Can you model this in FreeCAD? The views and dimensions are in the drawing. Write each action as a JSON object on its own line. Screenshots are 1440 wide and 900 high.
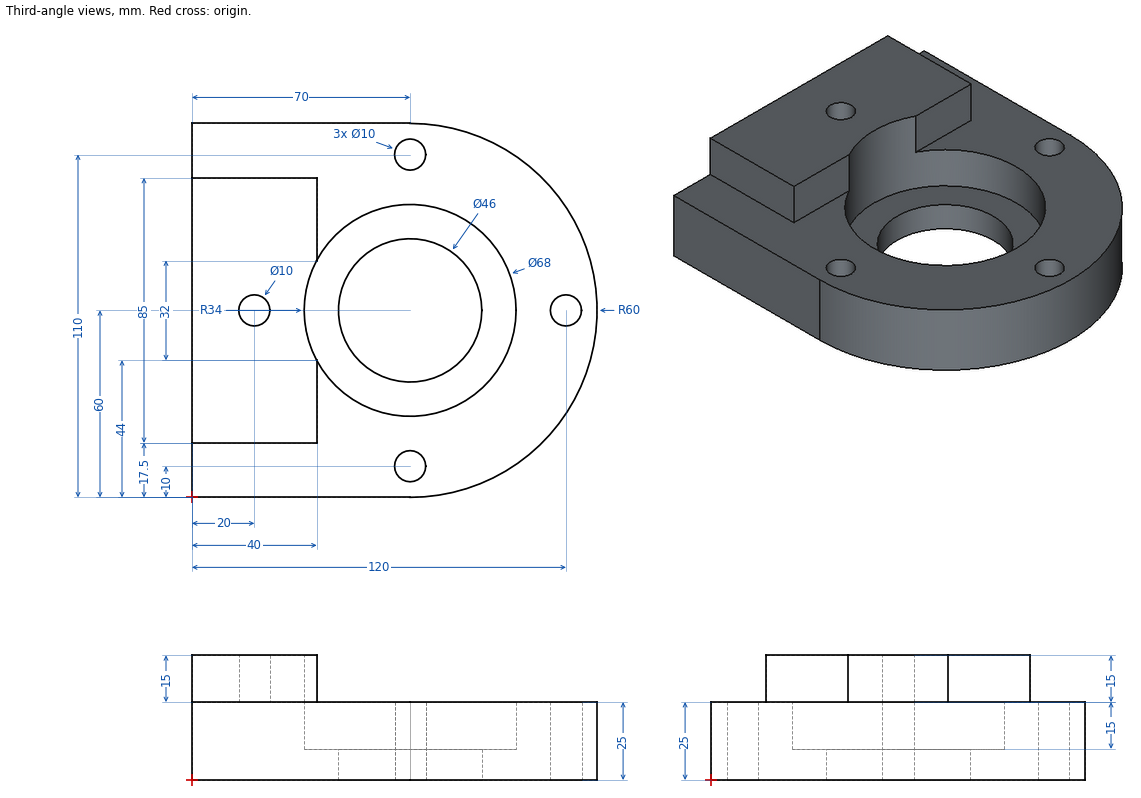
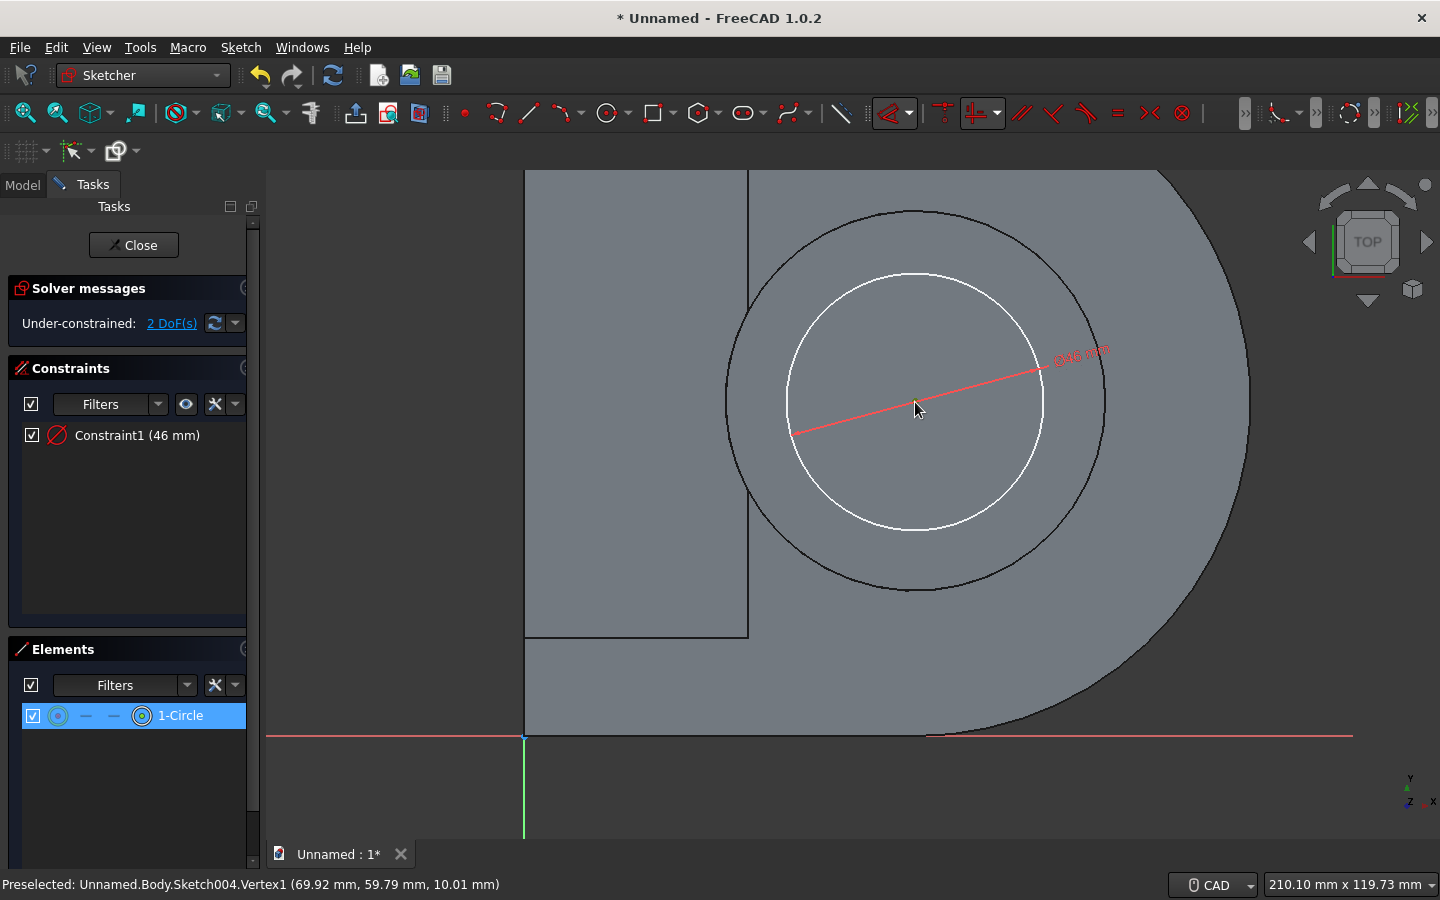
{"action": "key", "text": "l"}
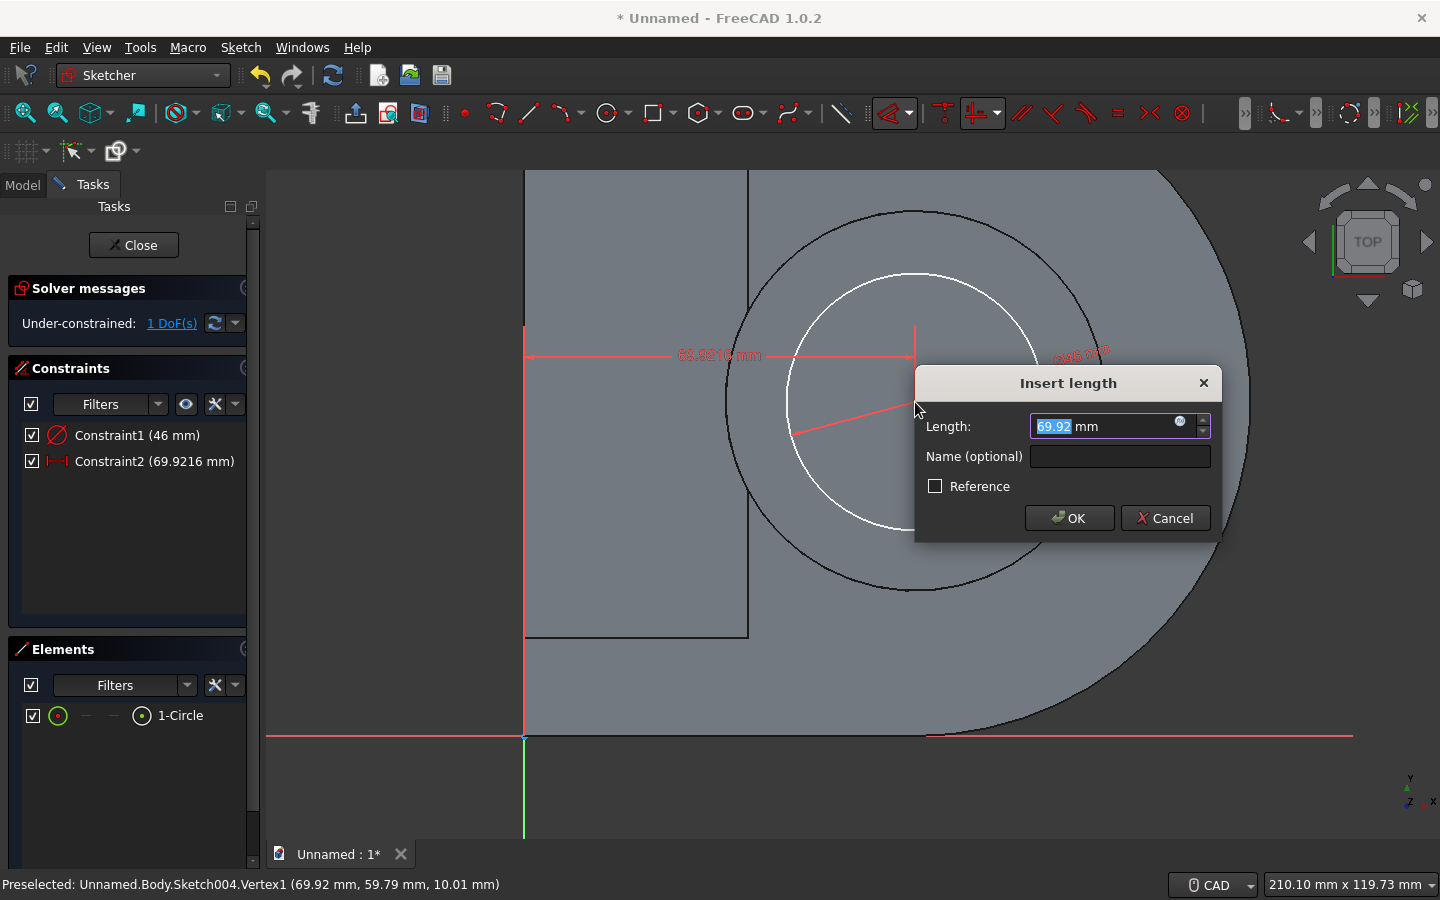
{"action": "type", "text": "70"}
{"action": "key", "text": "Return"}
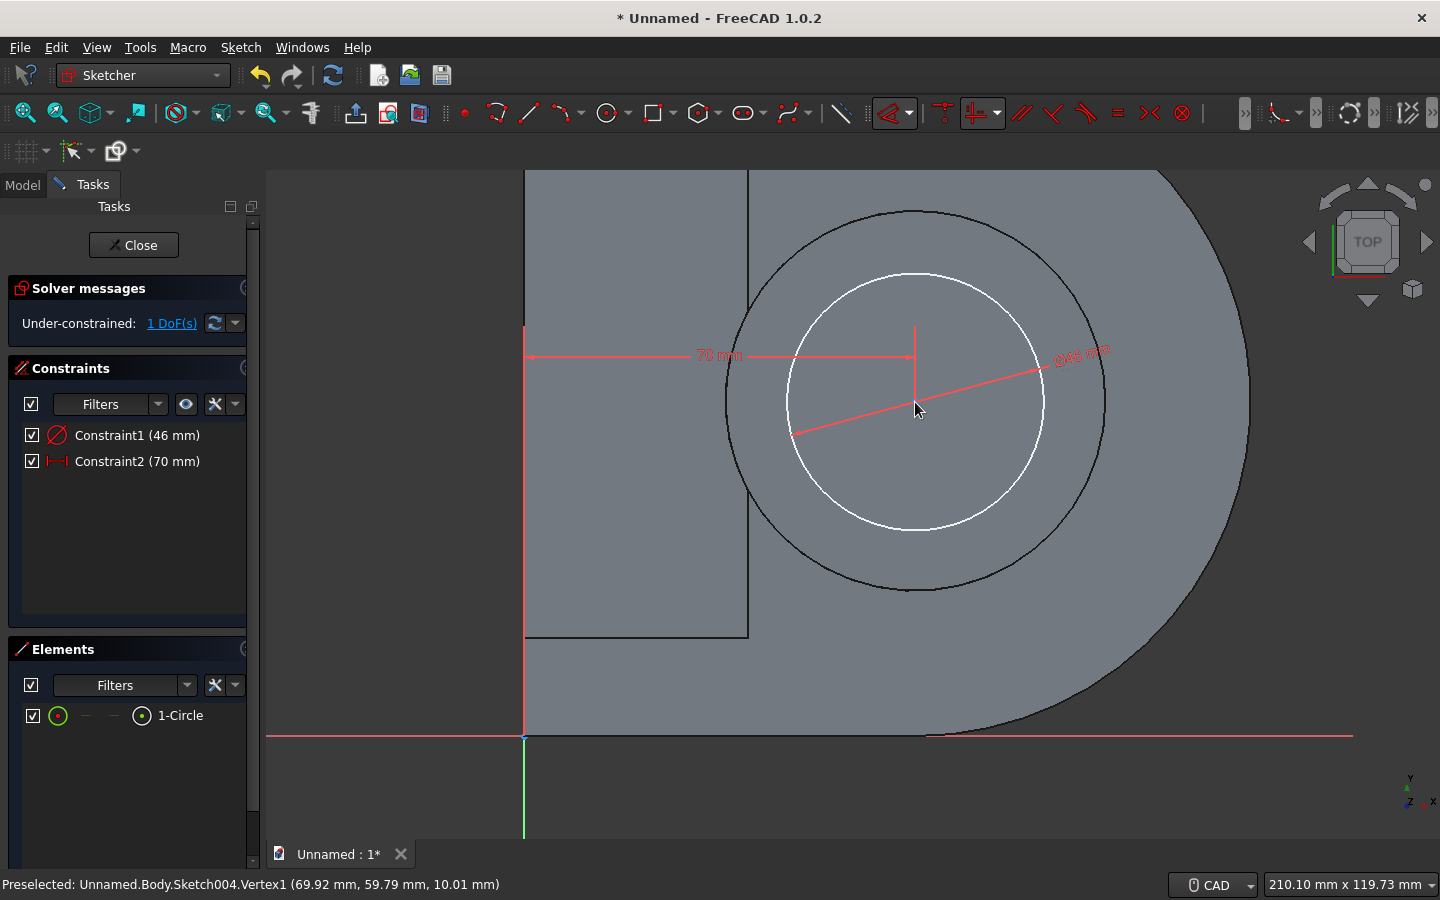
{"action": "left_click", "coordinate": [915, 402]}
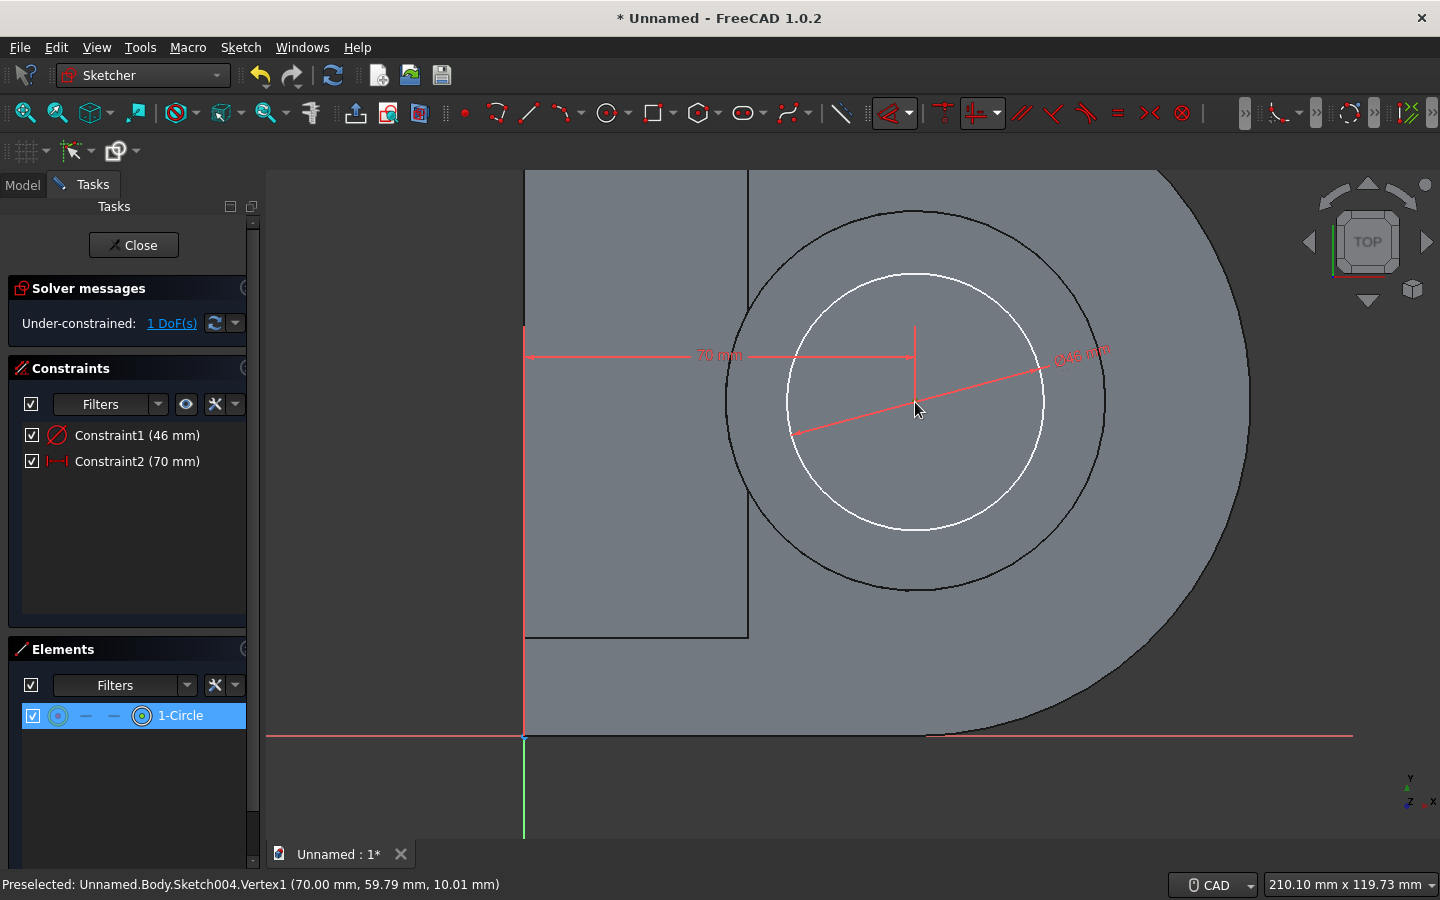
{"action": "left_click", "coordinate": [912, 114]}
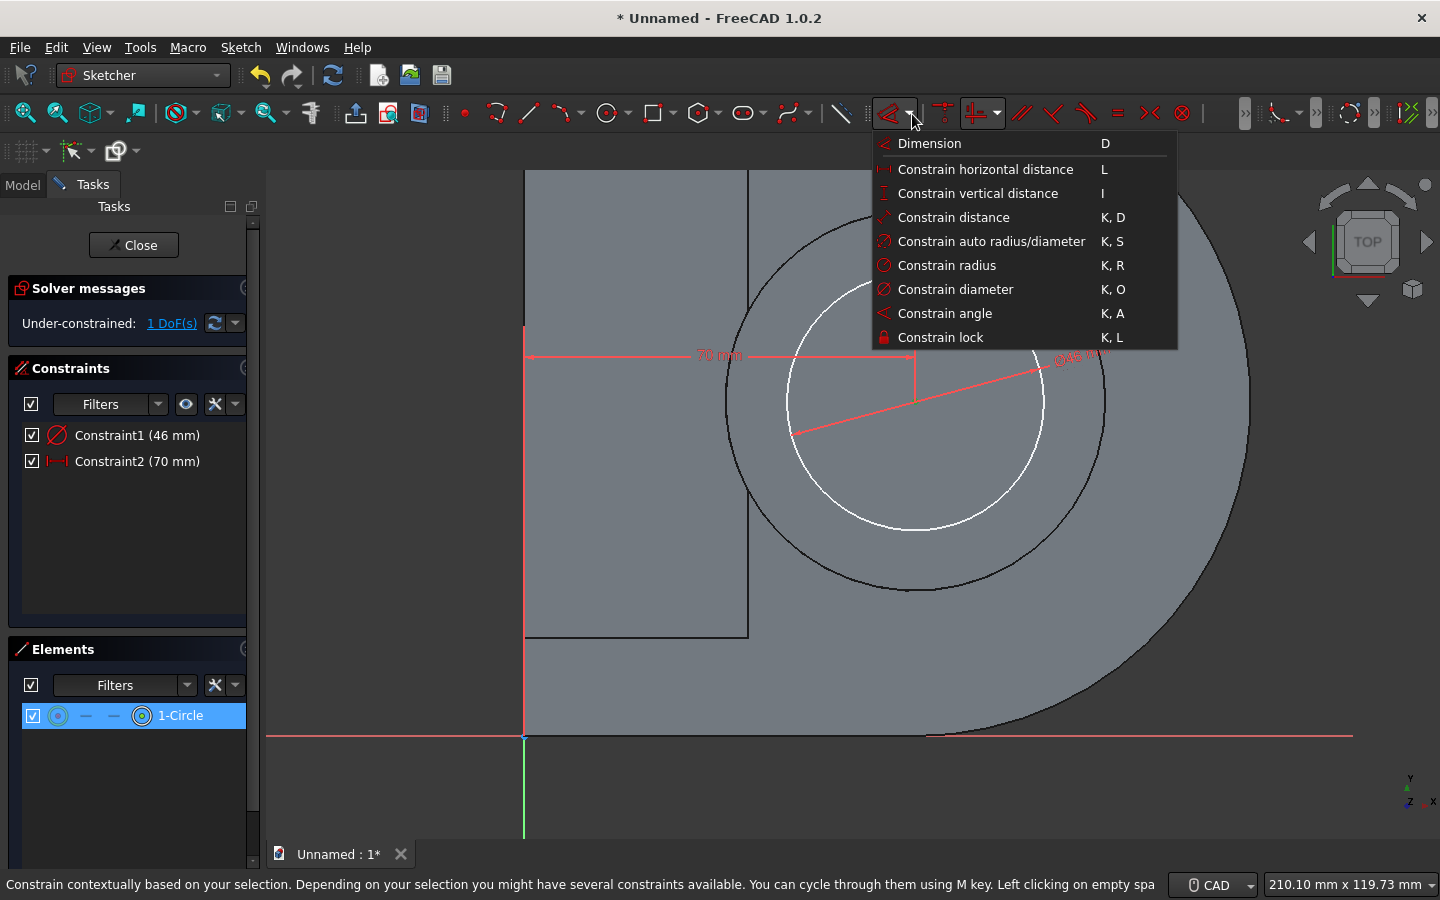
{"action": "left_click", "coordinate": [1025, 193]}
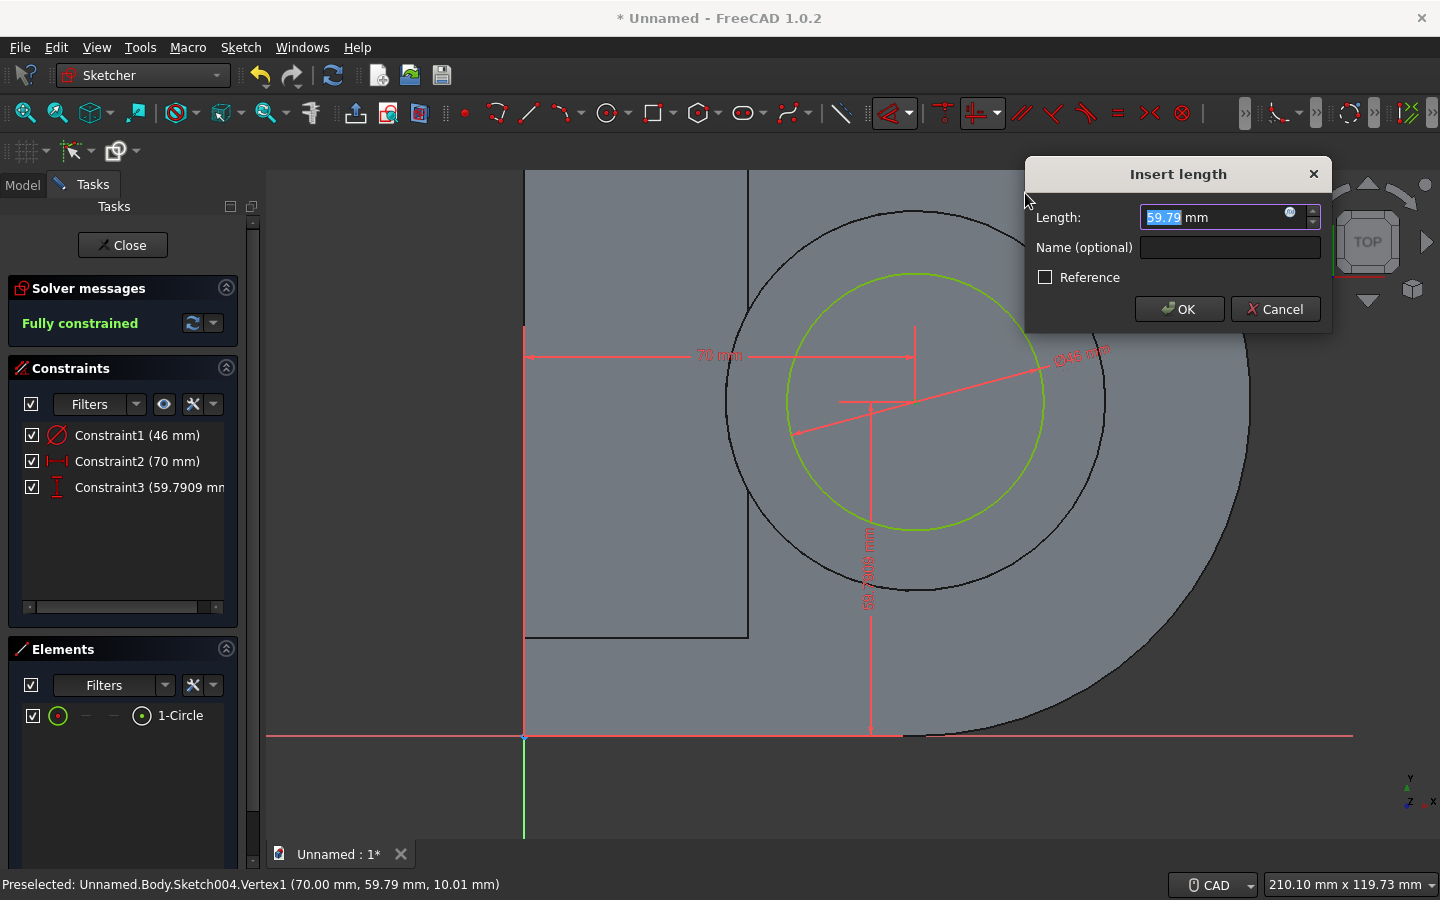
{"action": "type", "text": "60"}
{"action": "key", "text": "Return"}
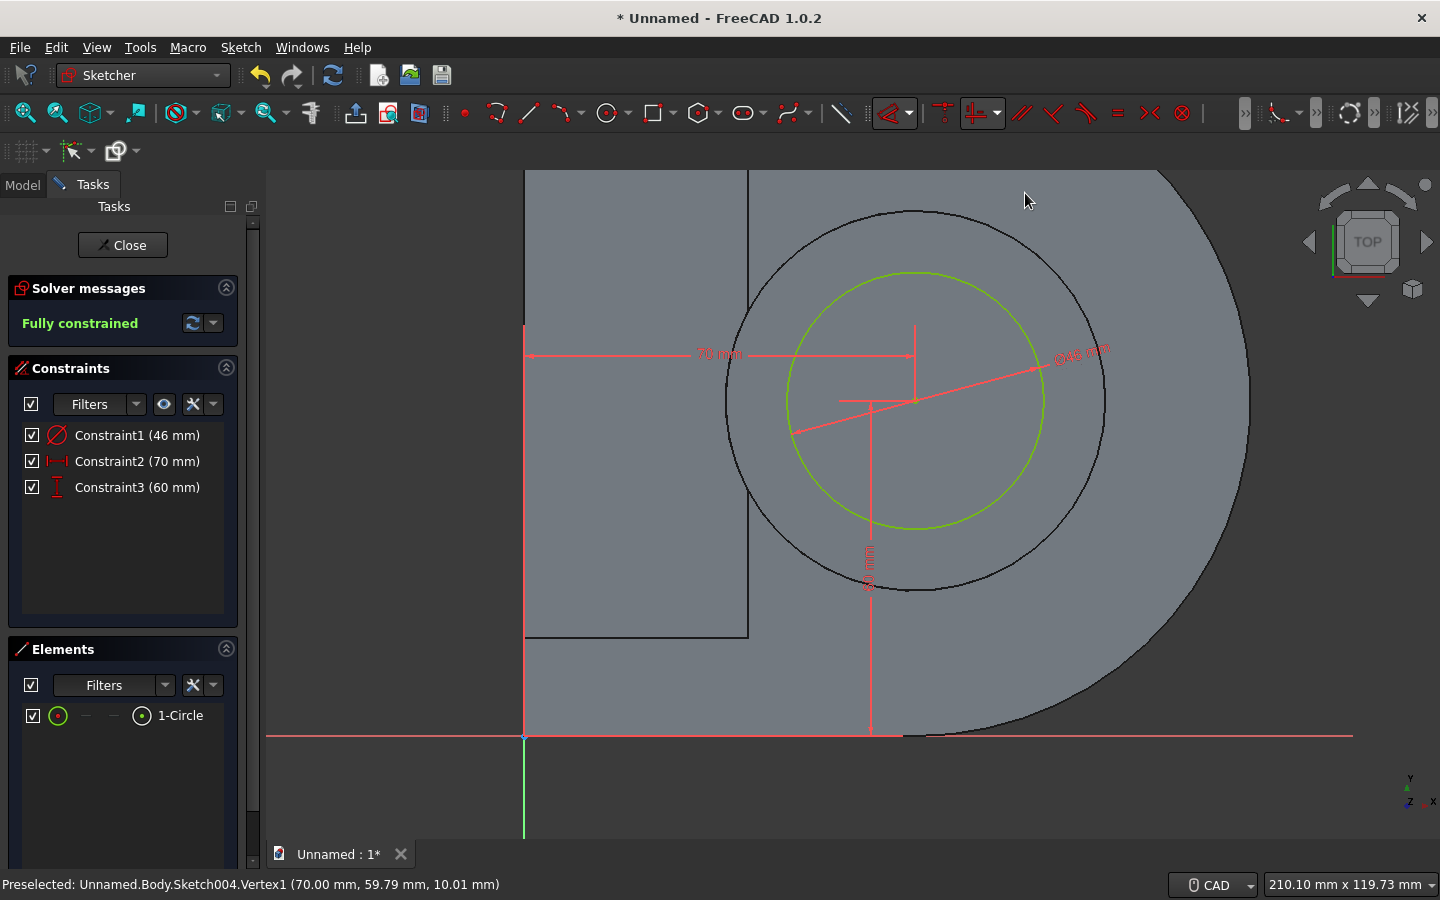
{"action": "left_click", "coordinate": [123, 245]}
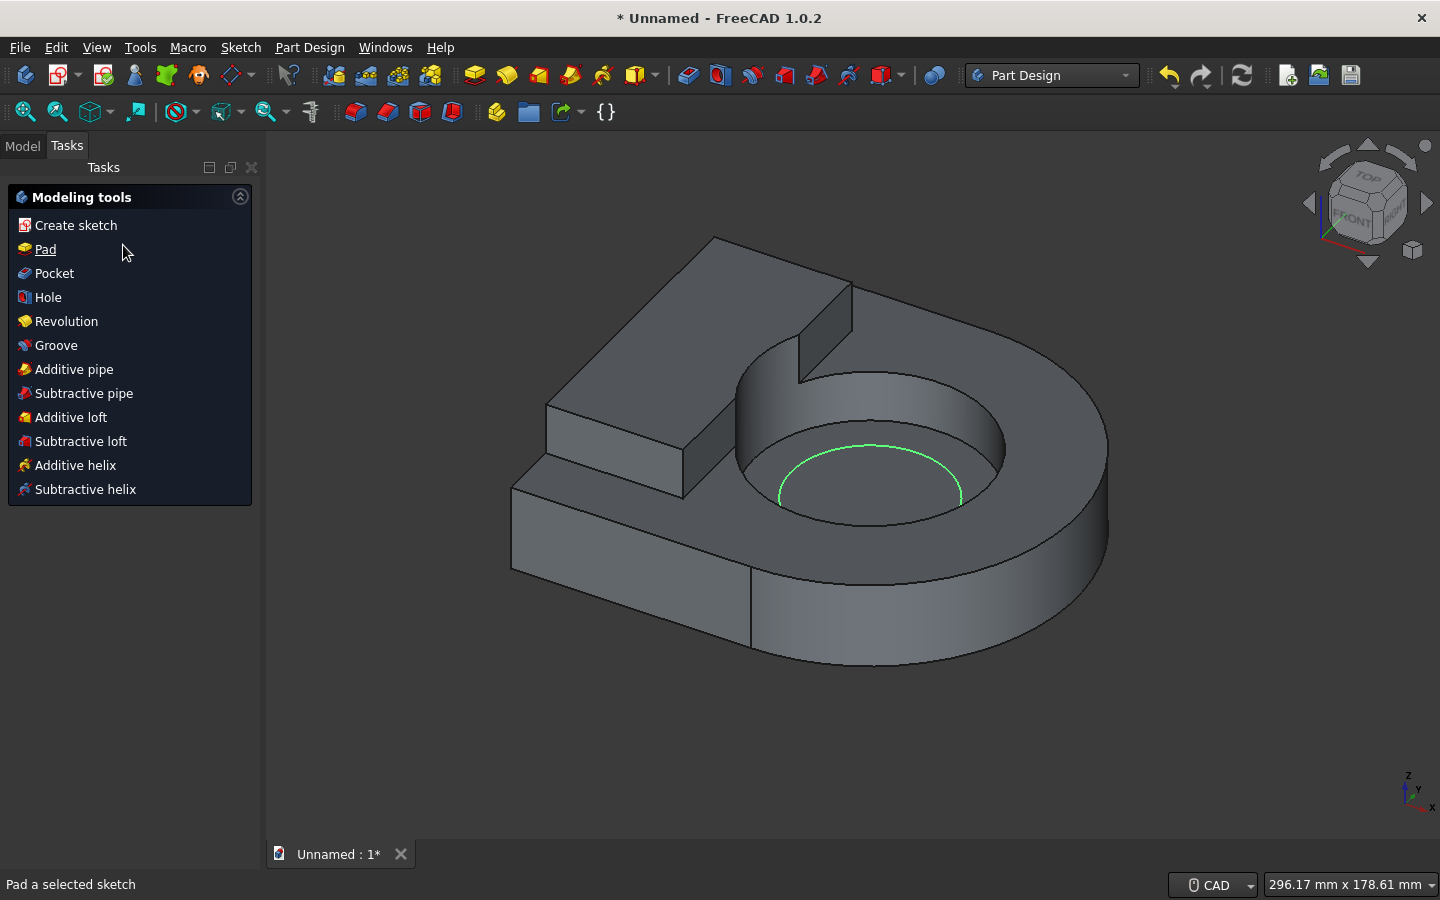
{"action": "left_click", "coordinate": [690, 76]}